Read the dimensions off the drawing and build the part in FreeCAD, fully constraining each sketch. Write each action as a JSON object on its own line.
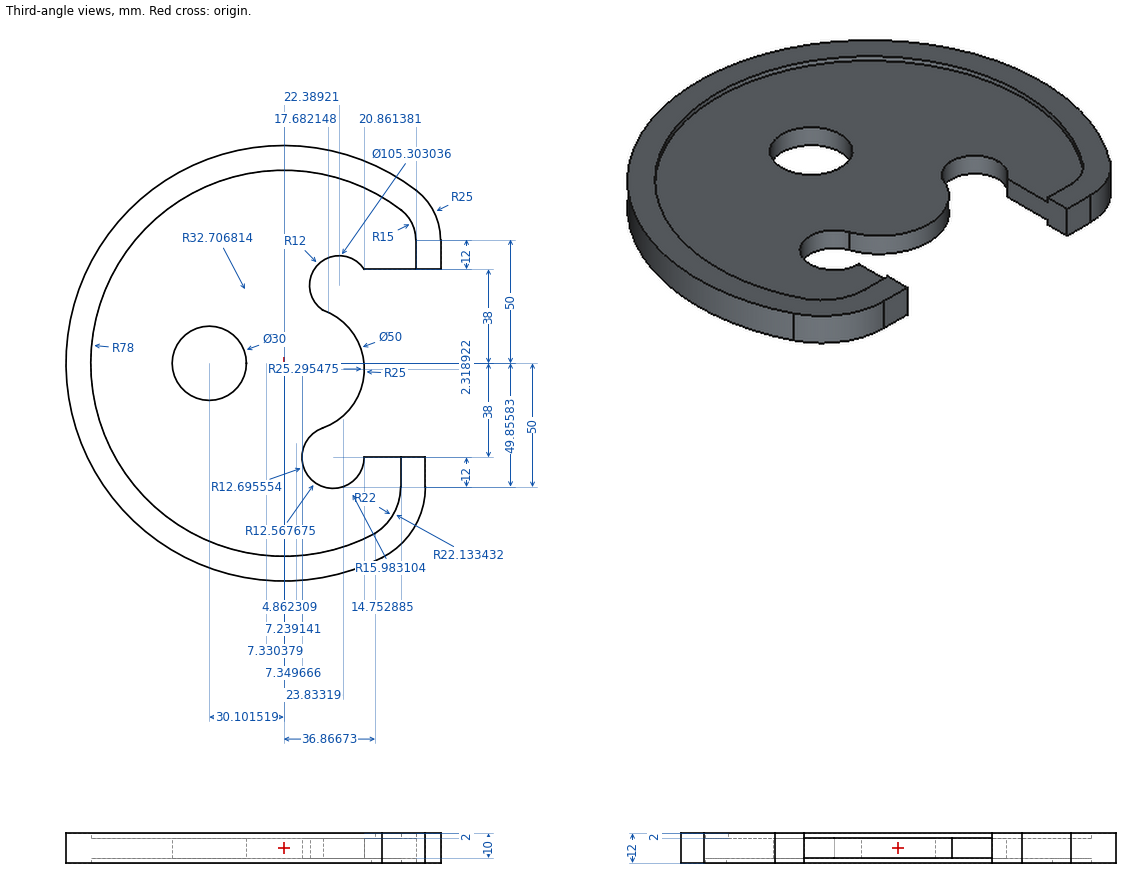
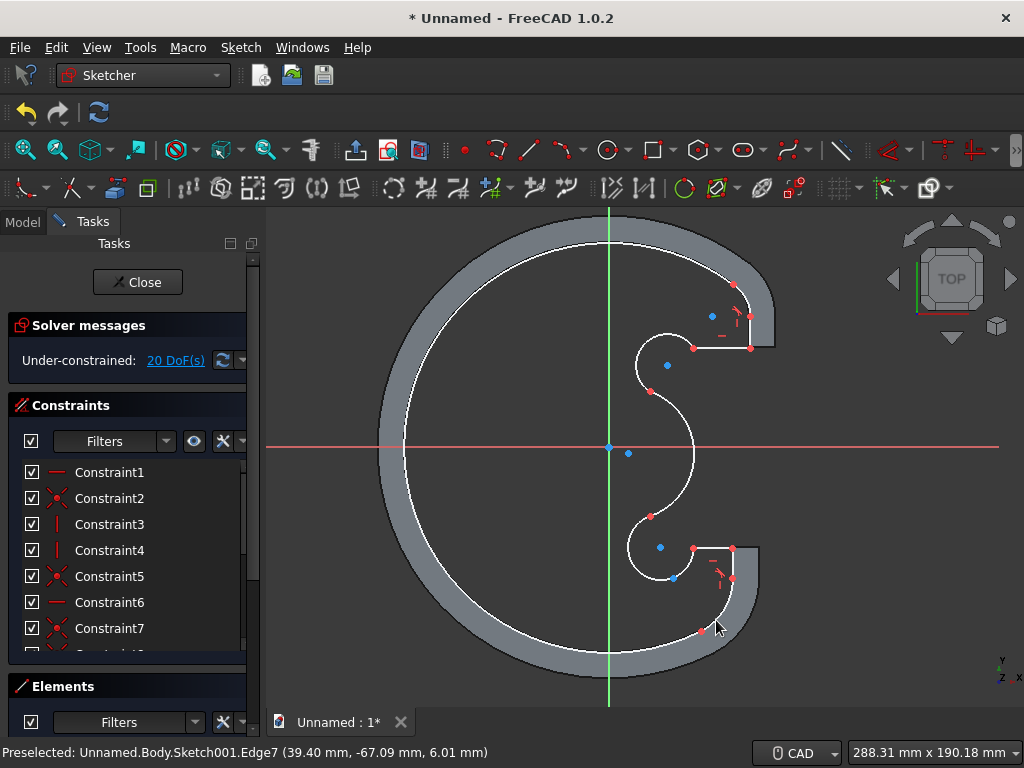
{"action": "scroll", "coordinate": [749, 305], "scroll_direction": "up", "scroll_amount": 2}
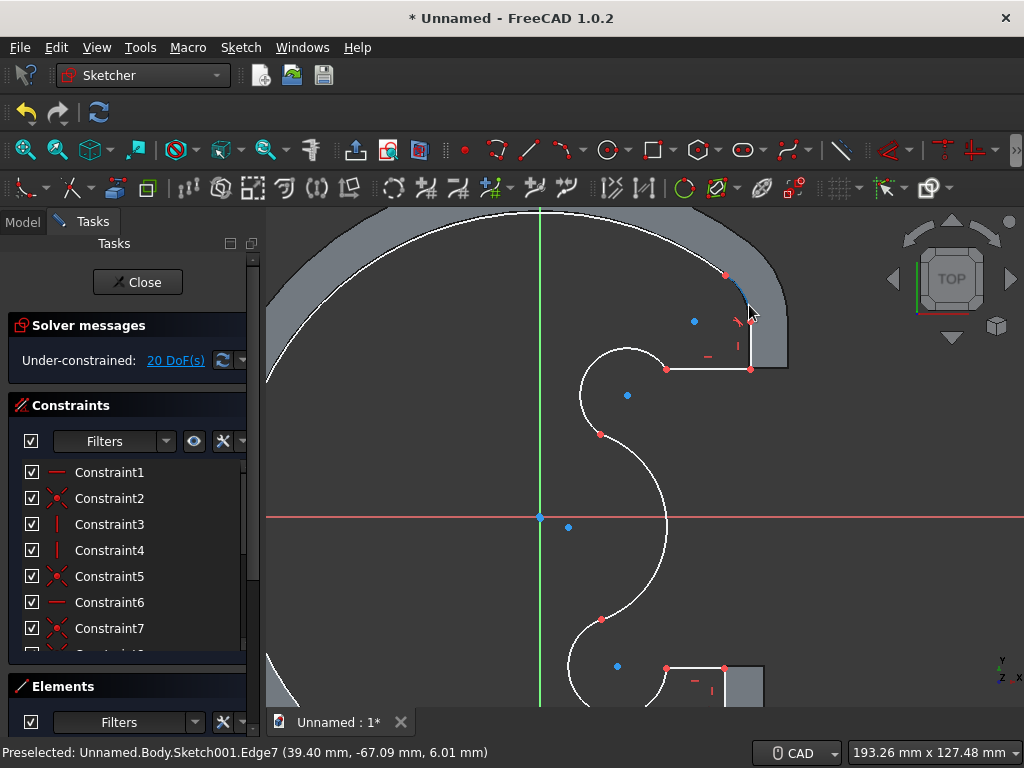
{"action": "left_click", "coordinate": [748, 305]}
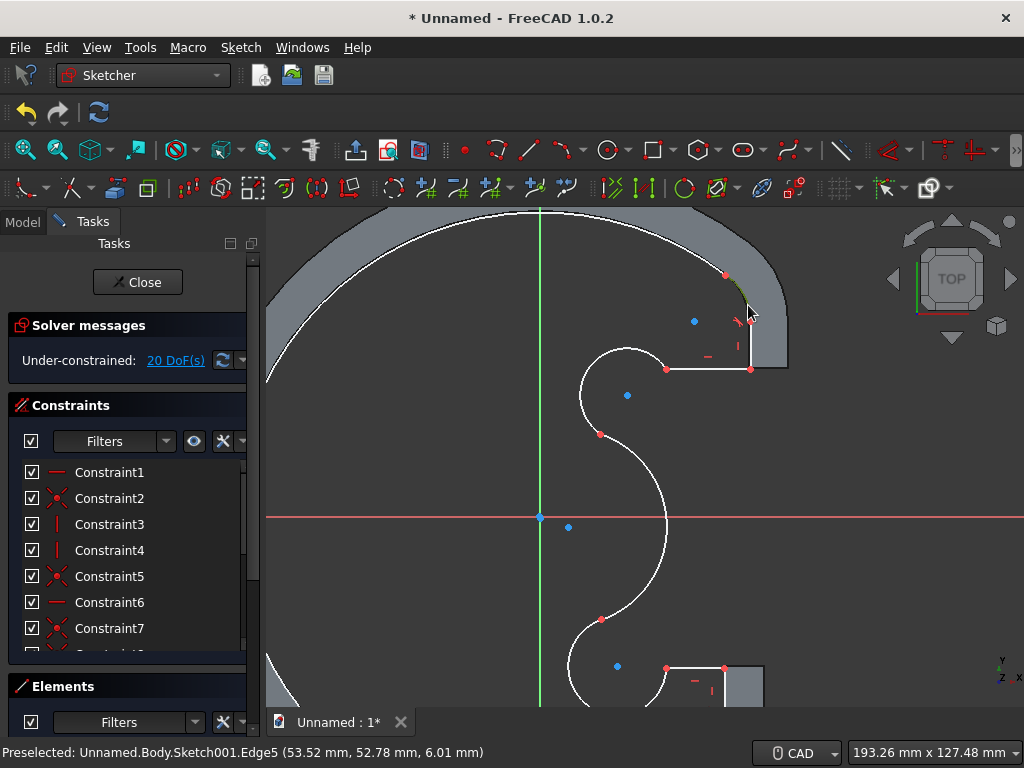
{"action": "left_click", "coordinate": [361, 270]}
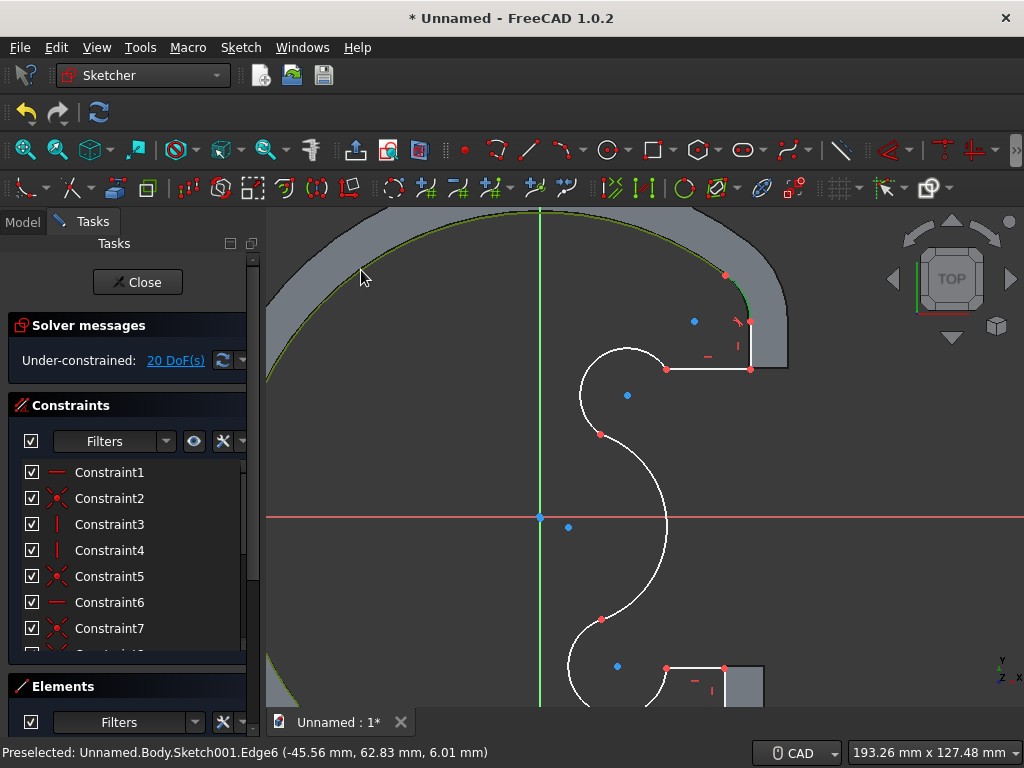
{"action": "key", "text": "t"}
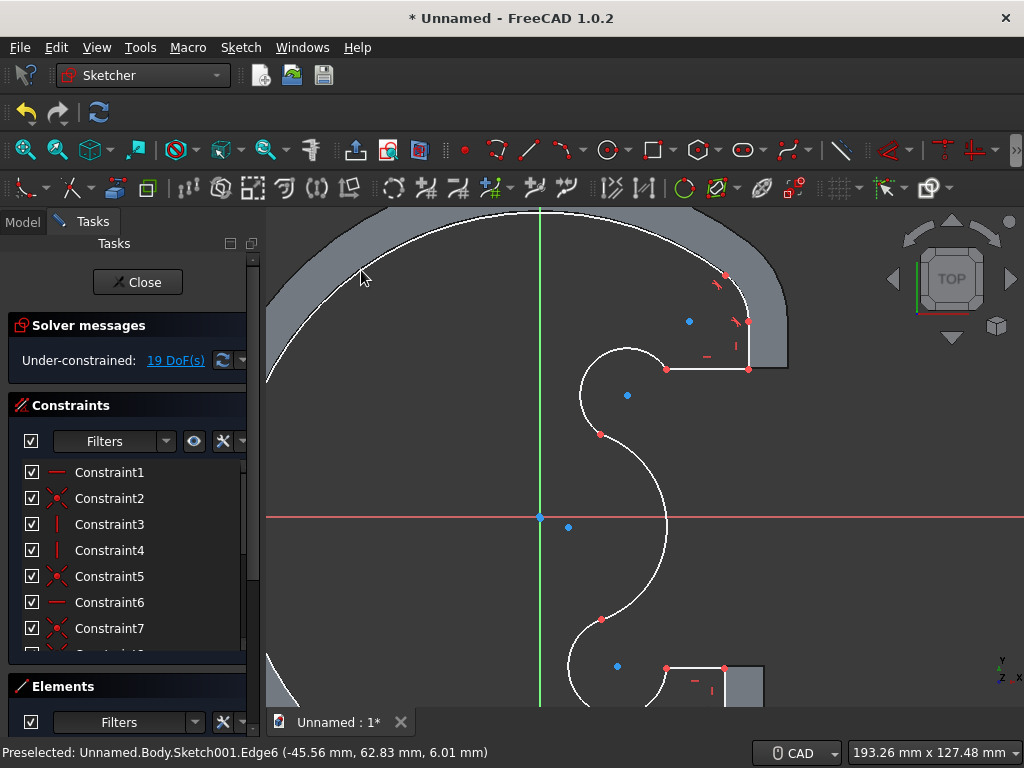
{"action": "left_click", "coordinate": [361, 270]}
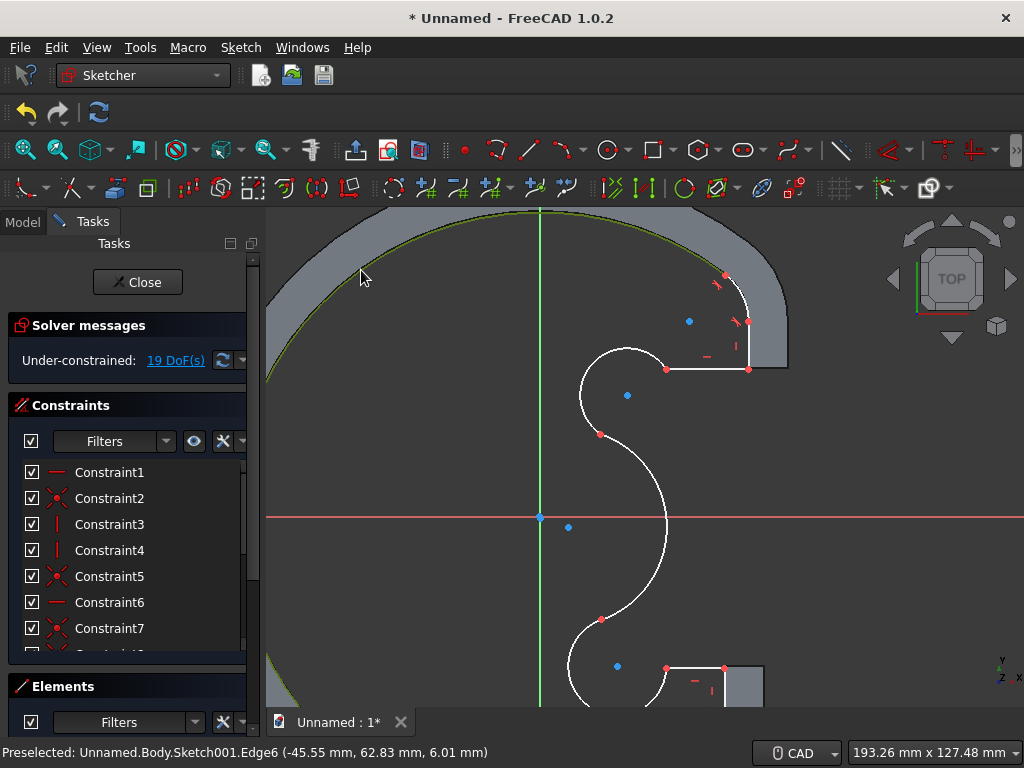
{"action": "scroll", "coordinate": [749, 305], "scroll_direction": "down", "scroll_amount": 2}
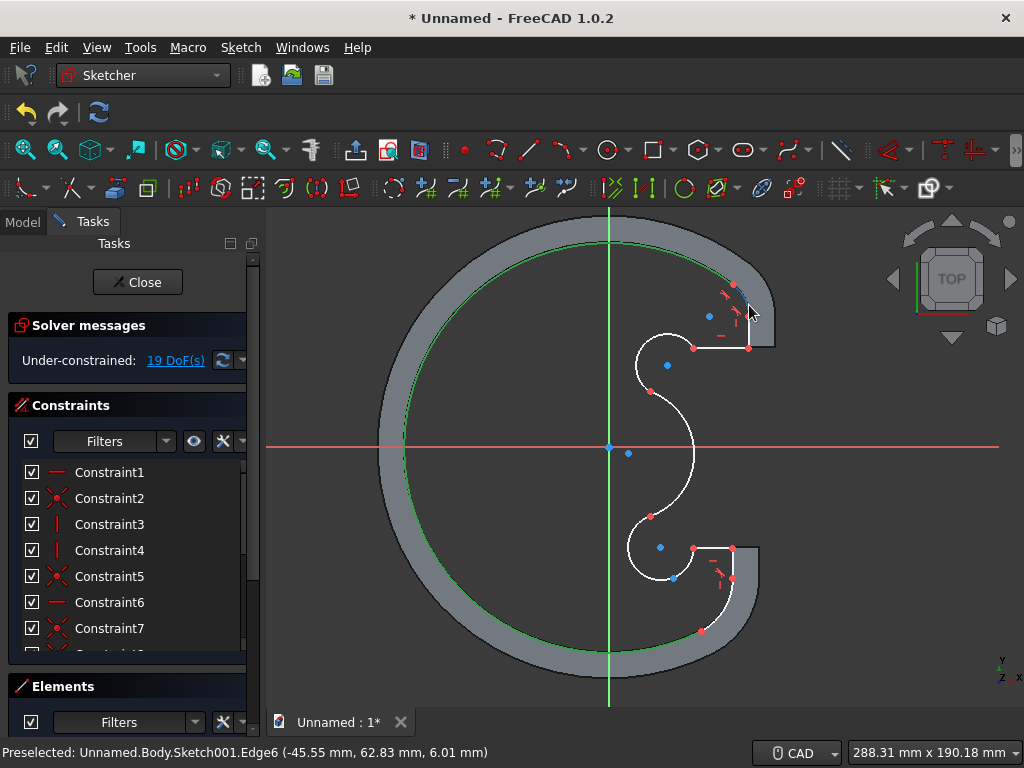
{"action": "left_click", "coordinate": [716, 620]}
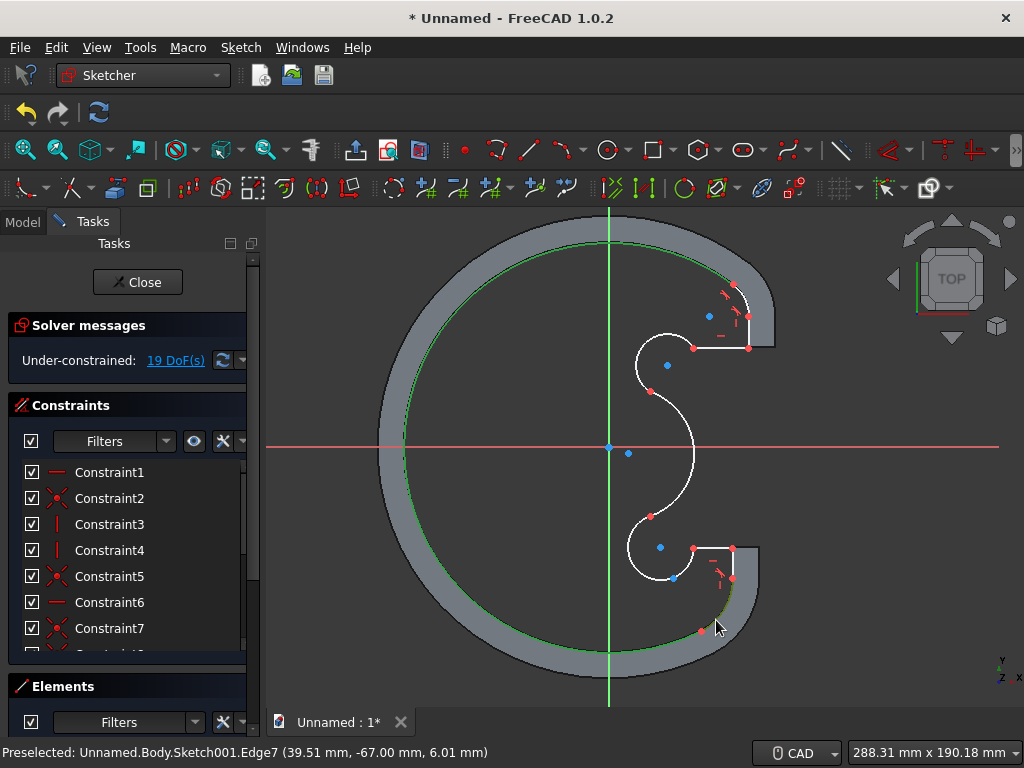
{"action": "key", "text": "t"}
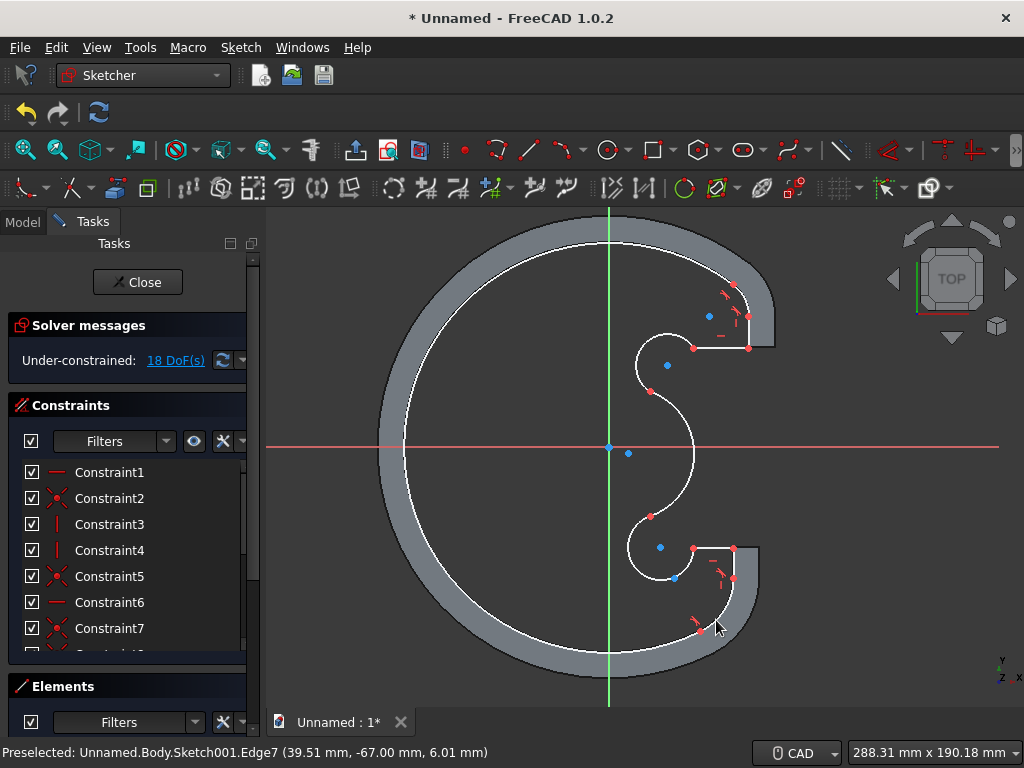
{"action": "left_click", "coordinate": [628, 549]}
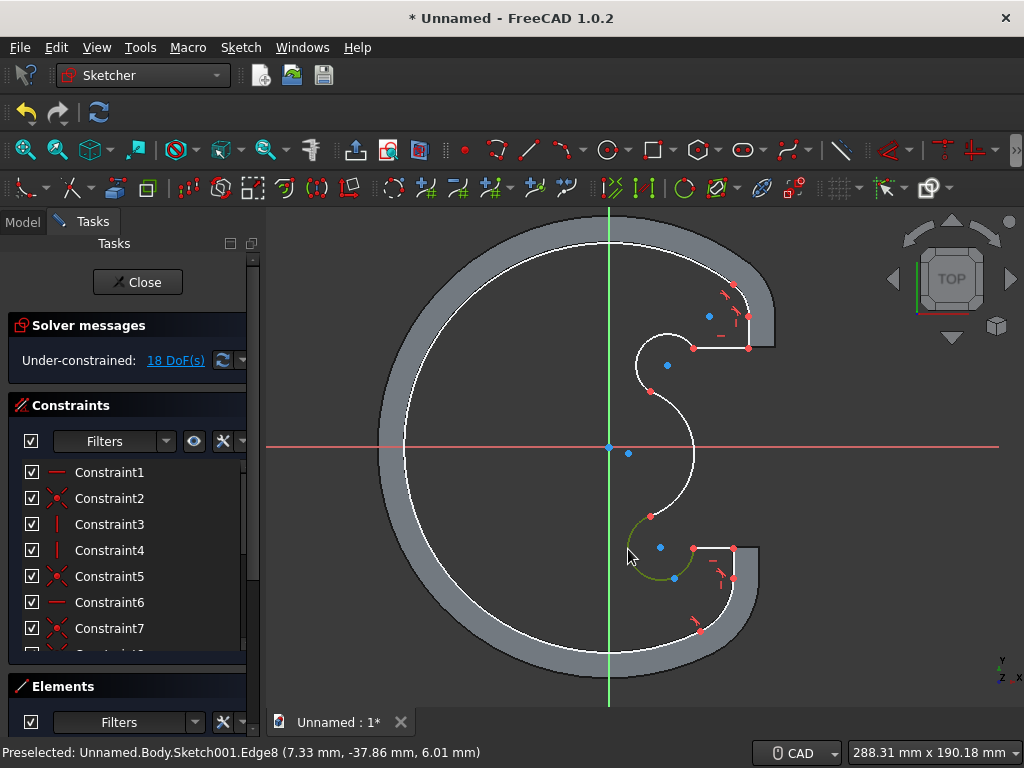
{"action": "left_click", "coordinate": [686, 485]}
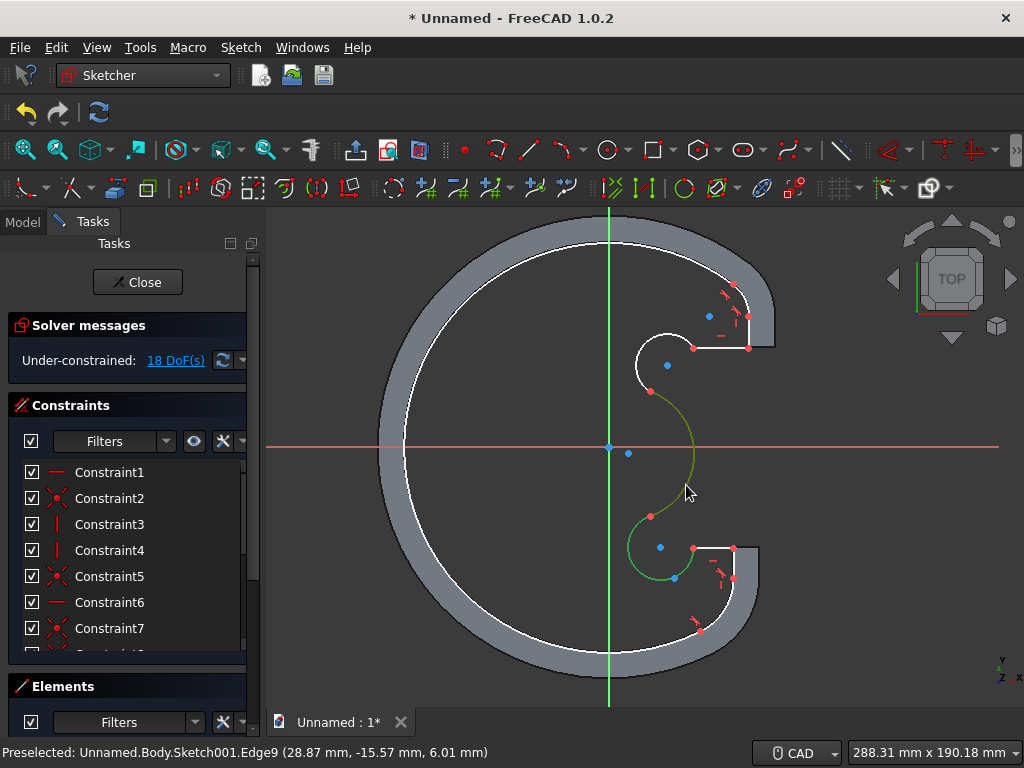
{"action": "key", "text": "t"}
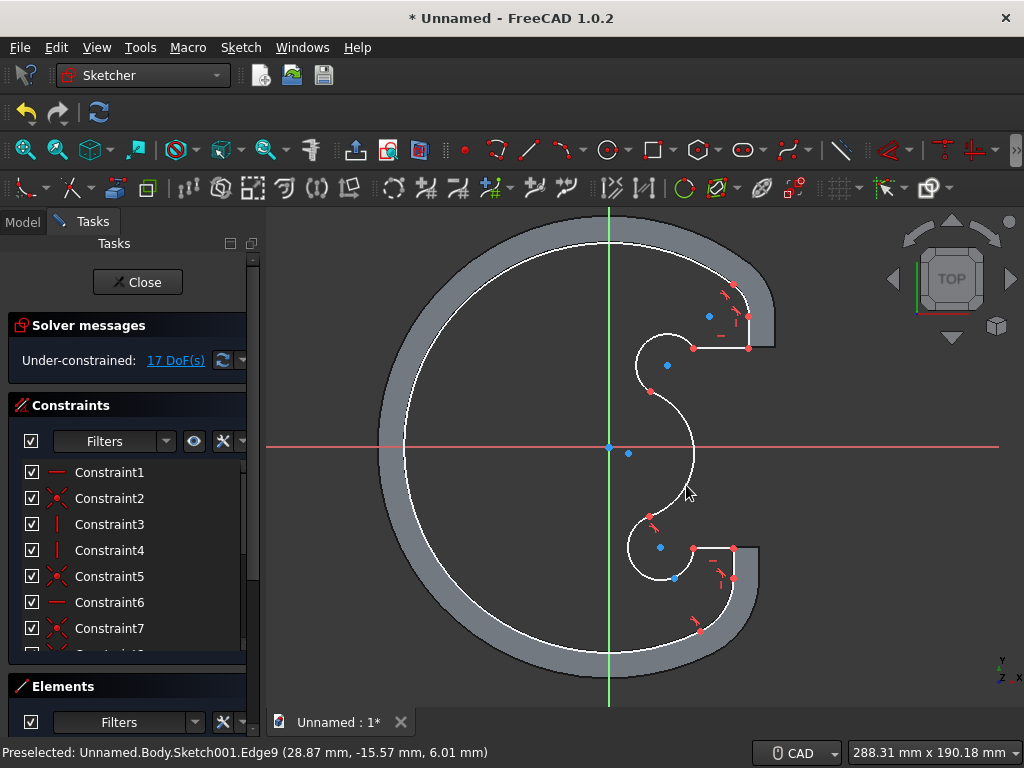
{"action": "scroll", "coordinate": [609, 447], "scroll_direction": "up", "scroll_amount": 2}